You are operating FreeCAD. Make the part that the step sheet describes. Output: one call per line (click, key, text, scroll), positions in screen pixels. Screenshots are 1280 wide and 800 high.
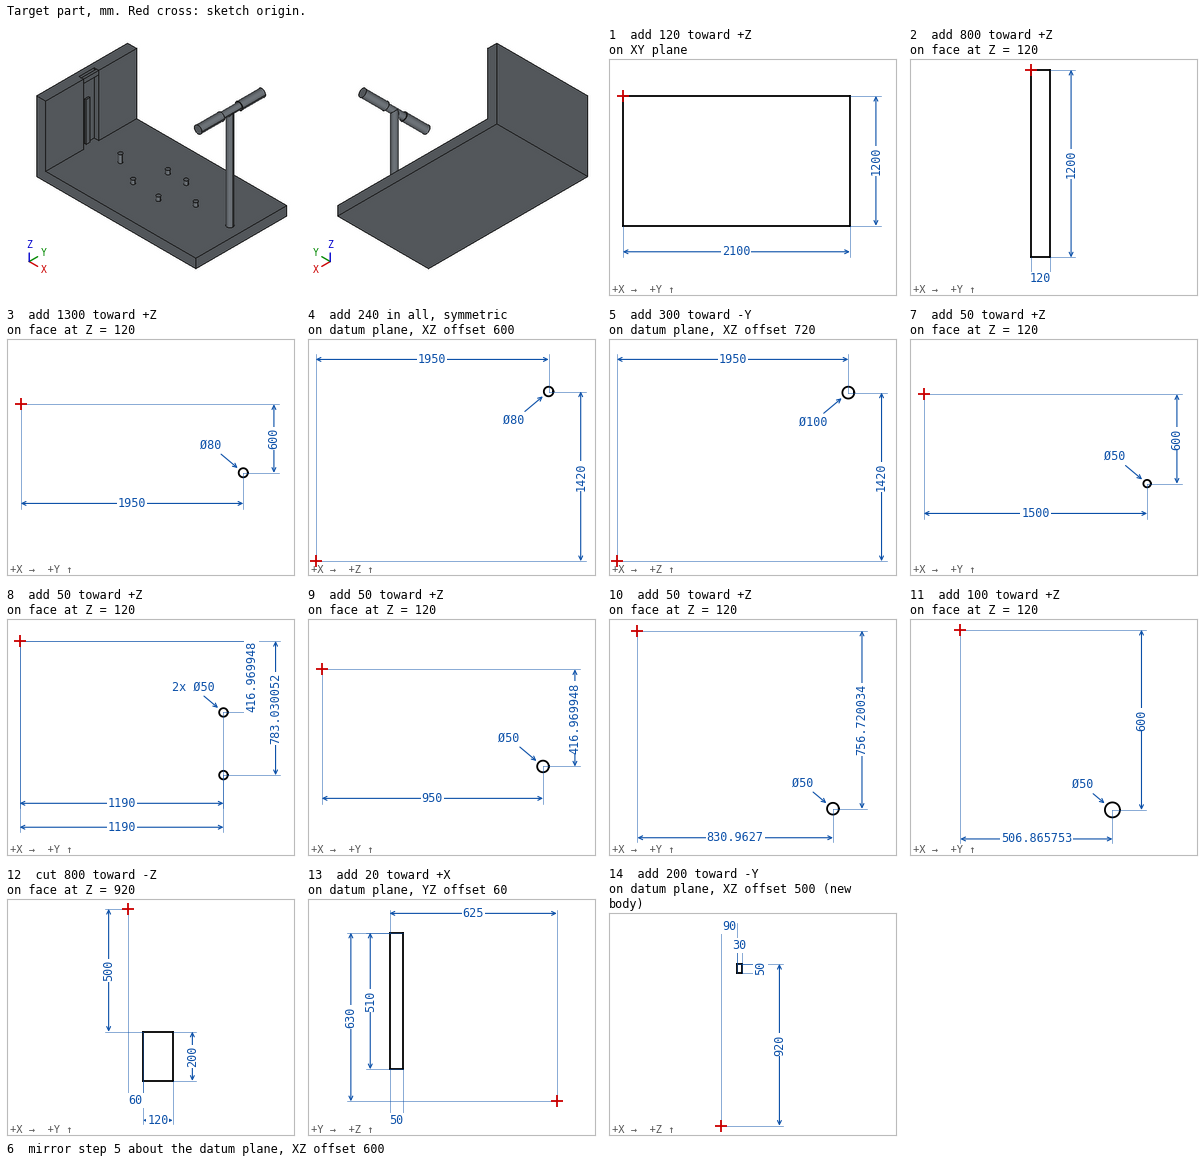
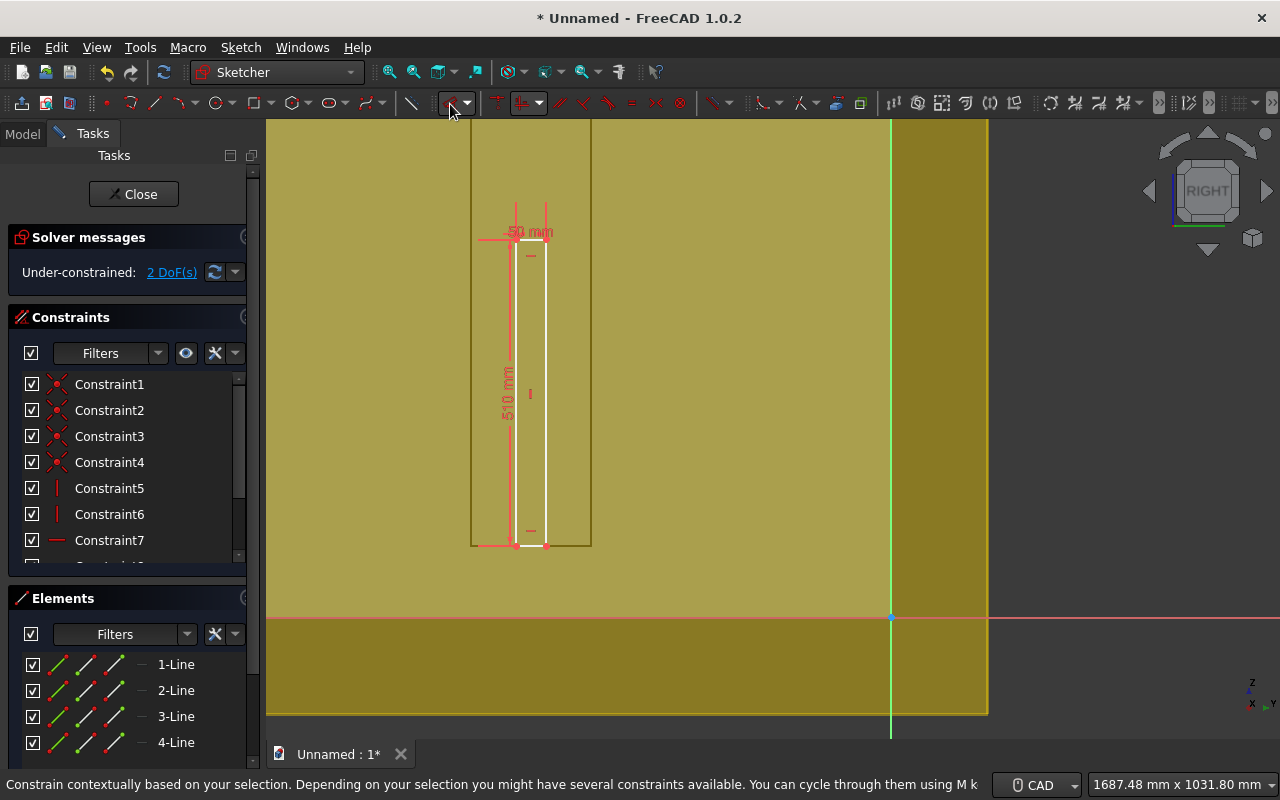
click(516, 240)
click(704, 652)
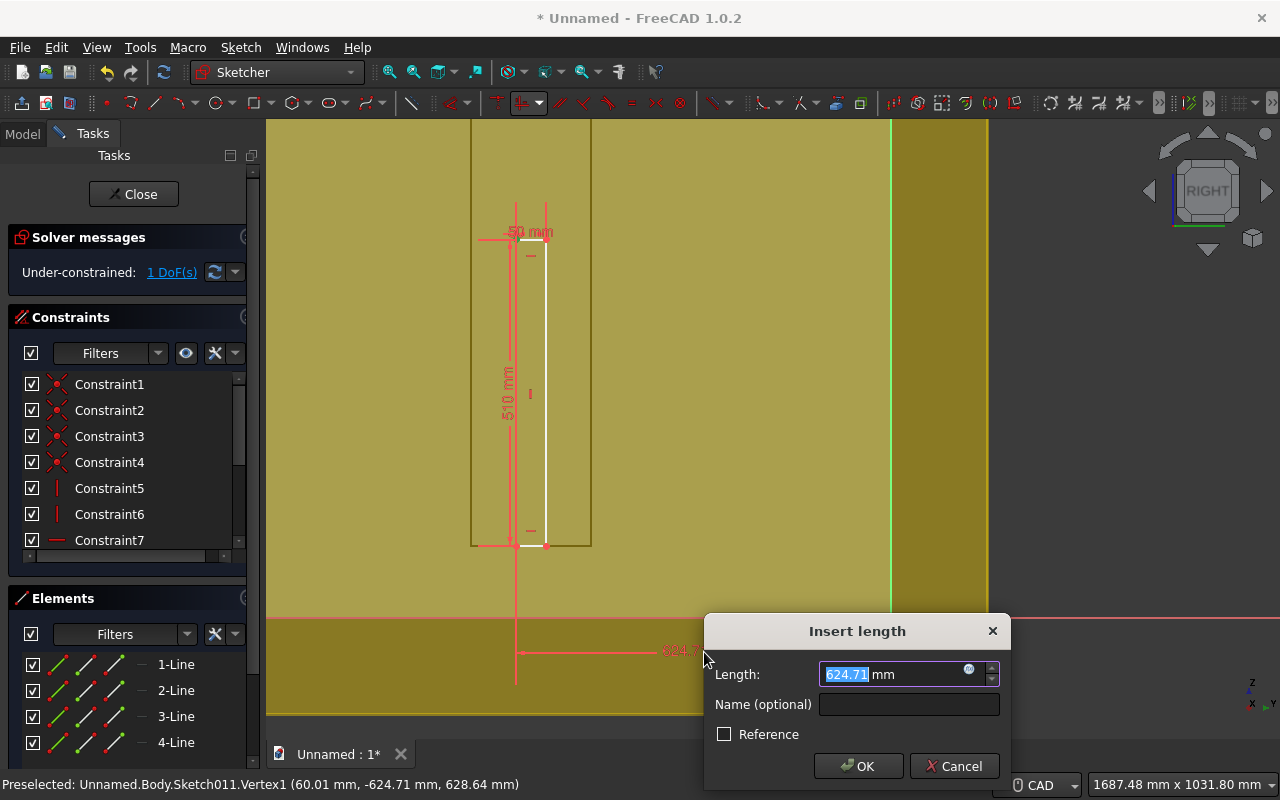
text(625)
key(Return)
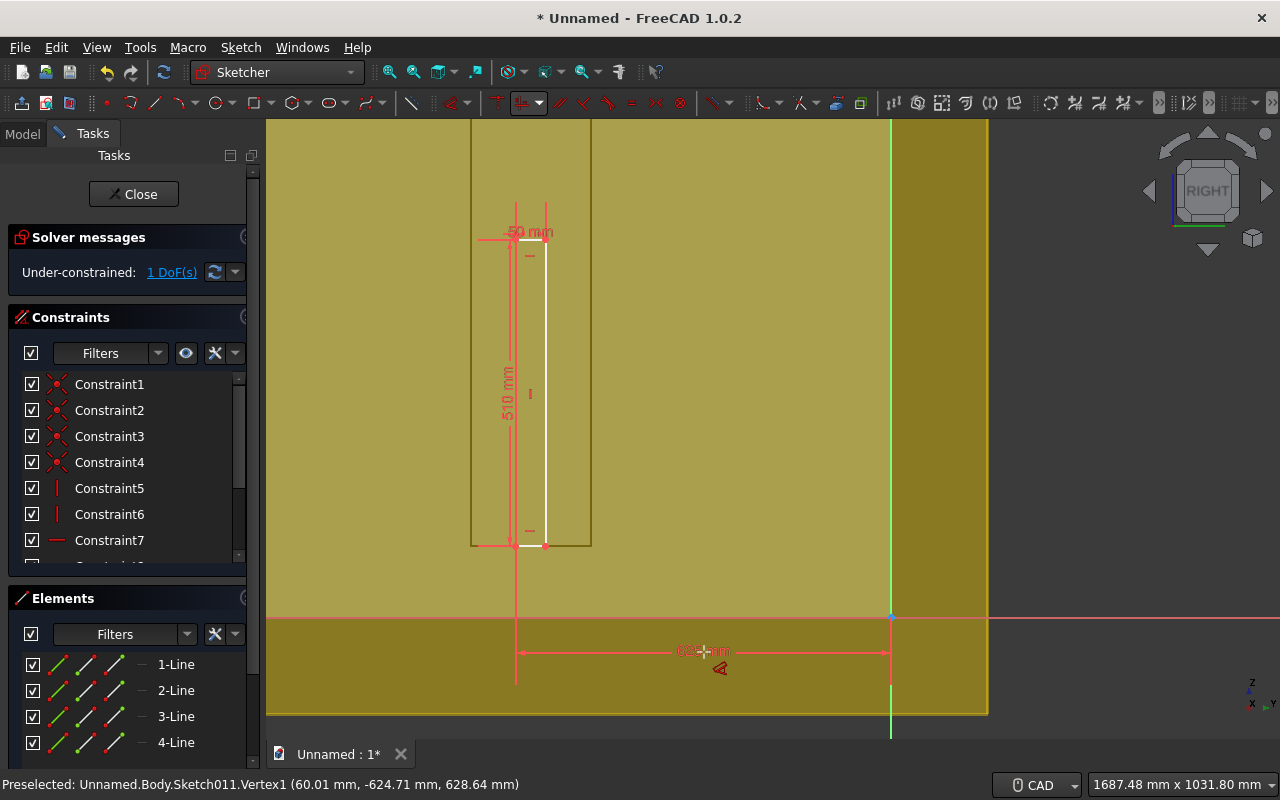
click(516, 240)
click(925, 429)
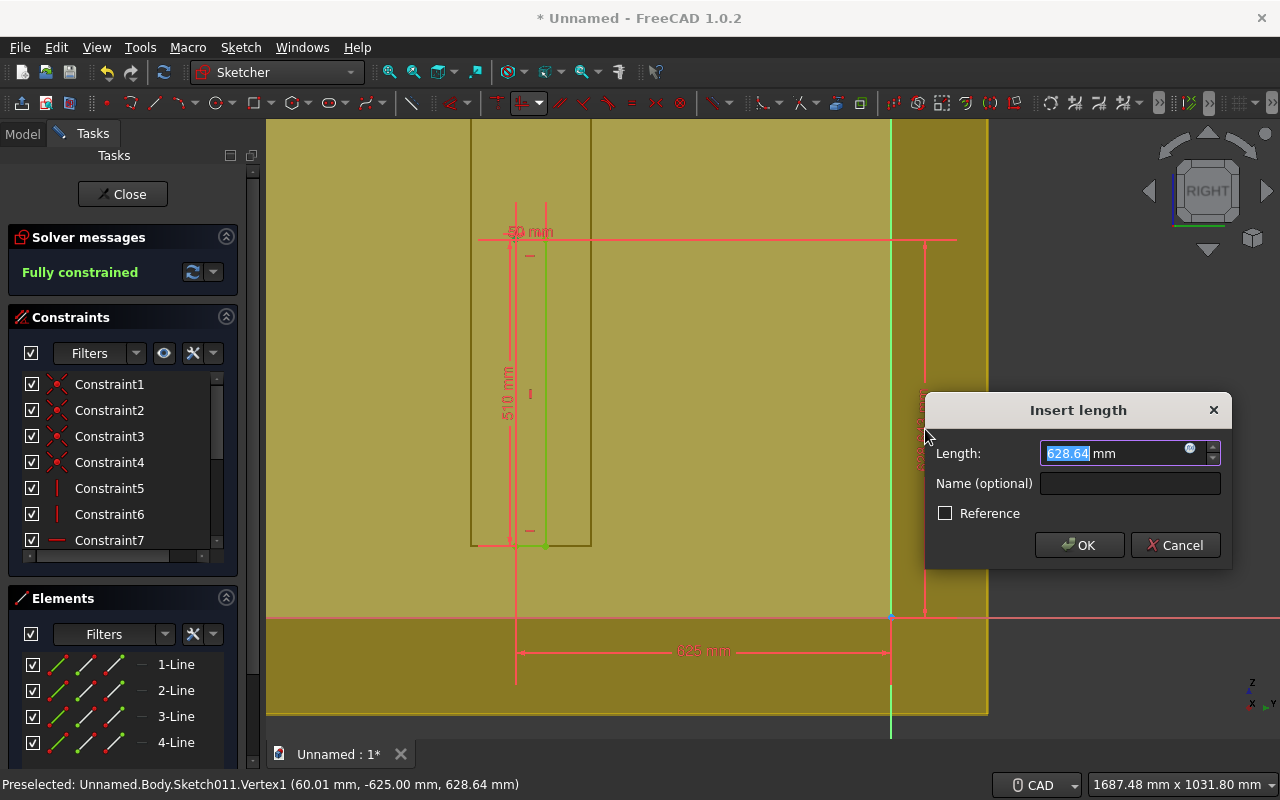
text(630)
key(Return)
key(Escape)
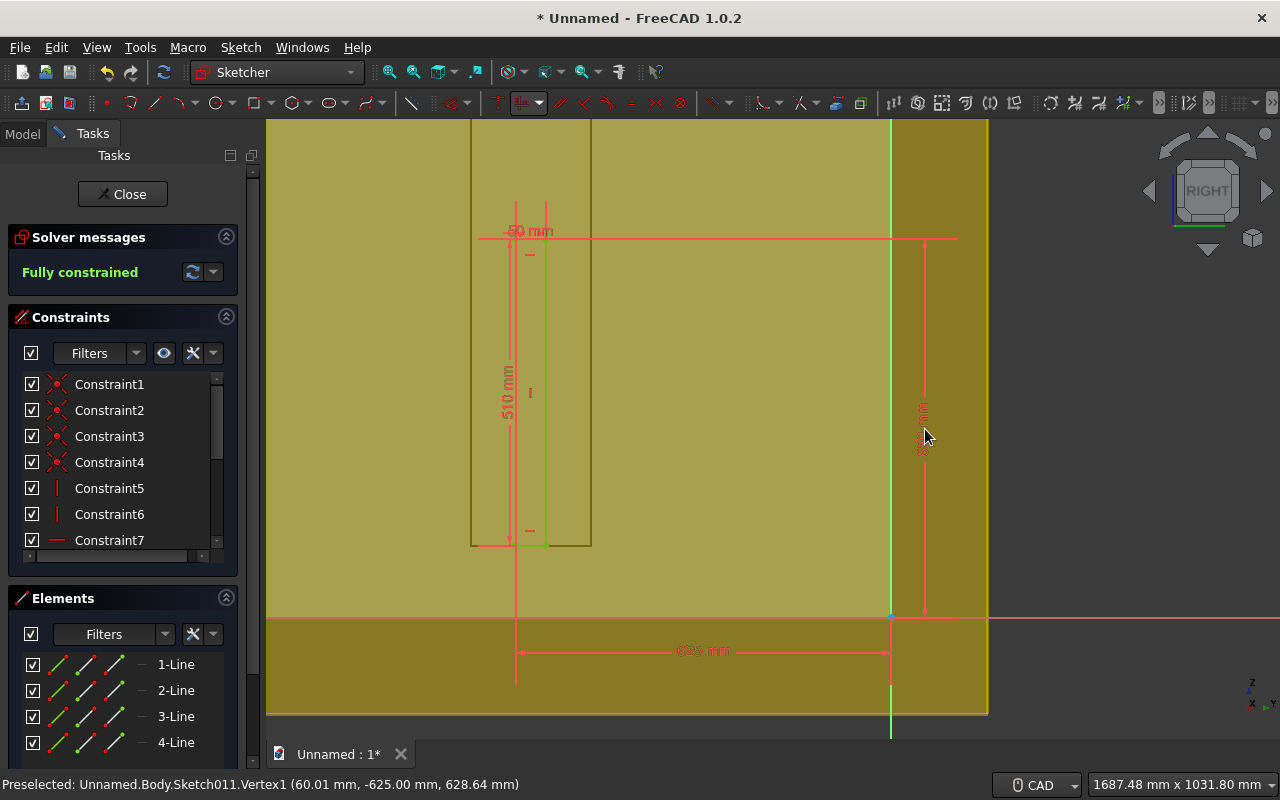
click(123, 194)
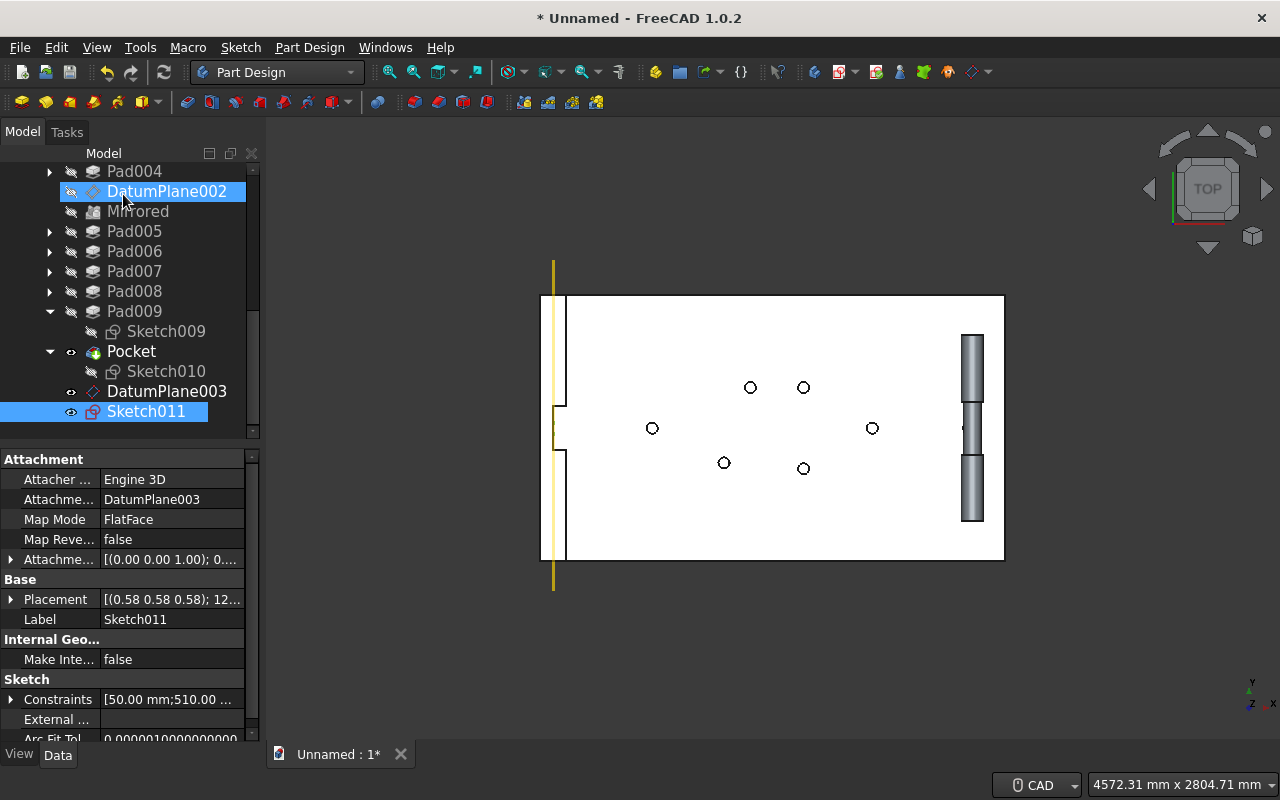
click(22, 102)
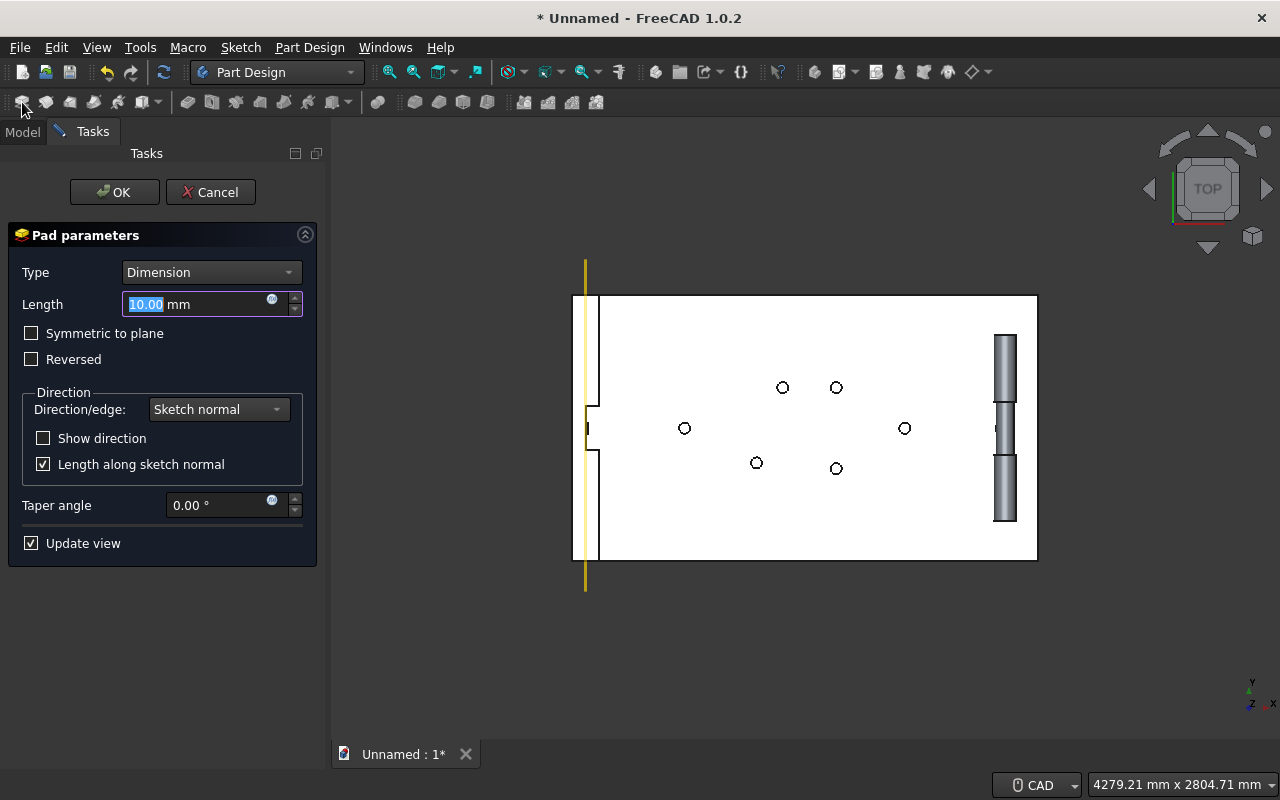
text(20)
key(Tab)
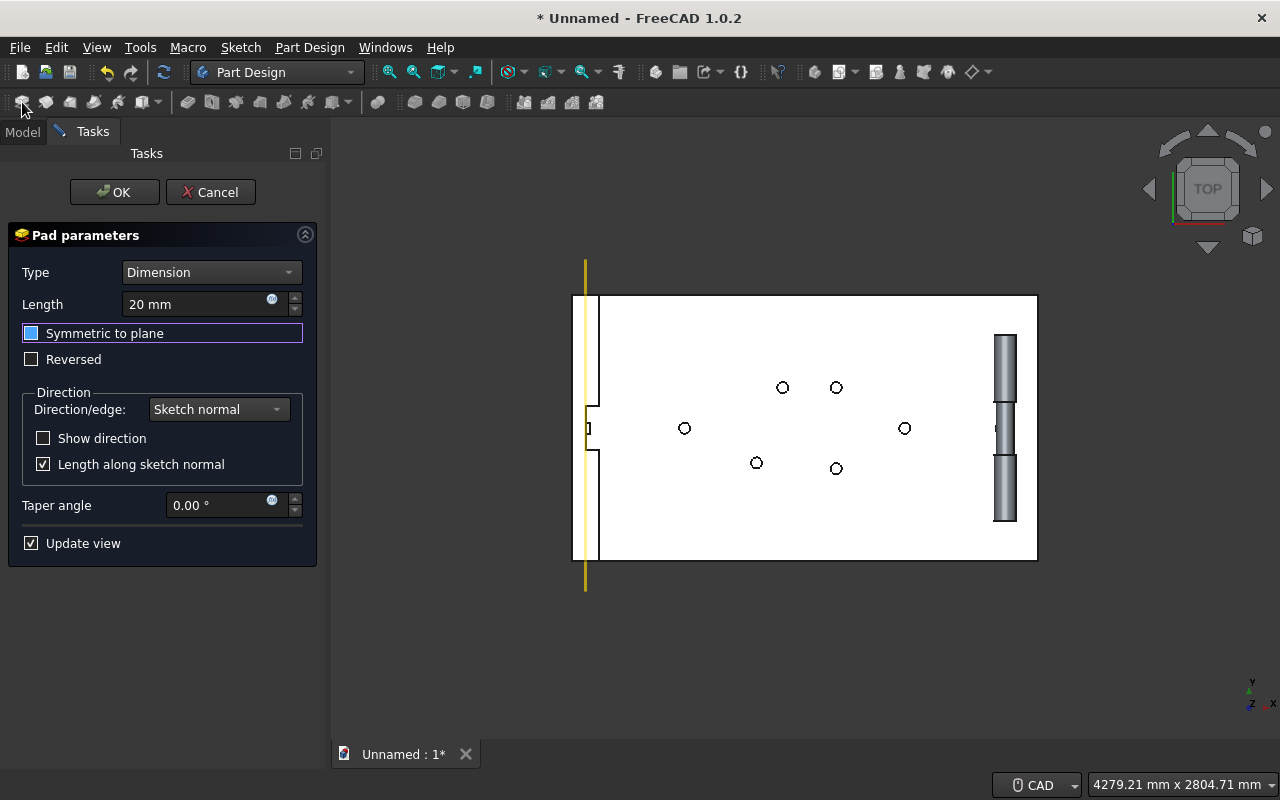
click(115, 192)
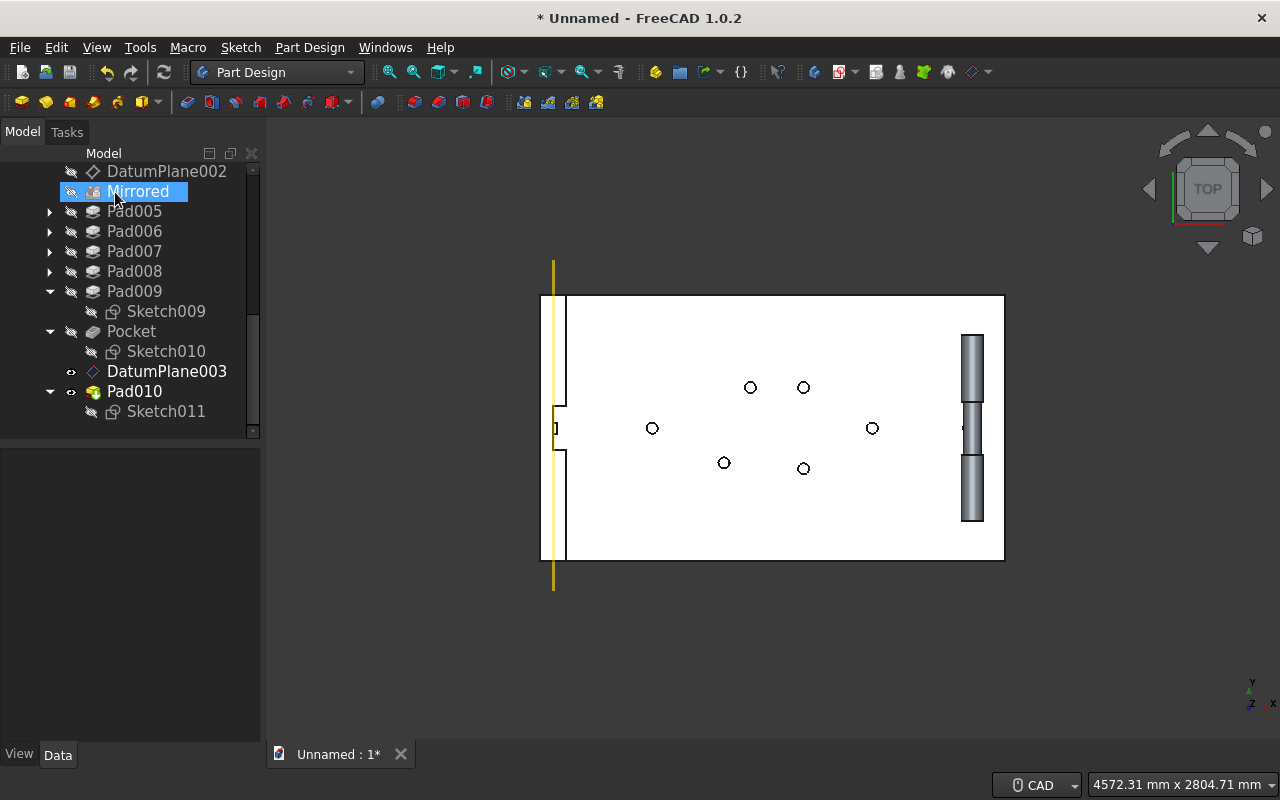
click(116, 372)
key(space)